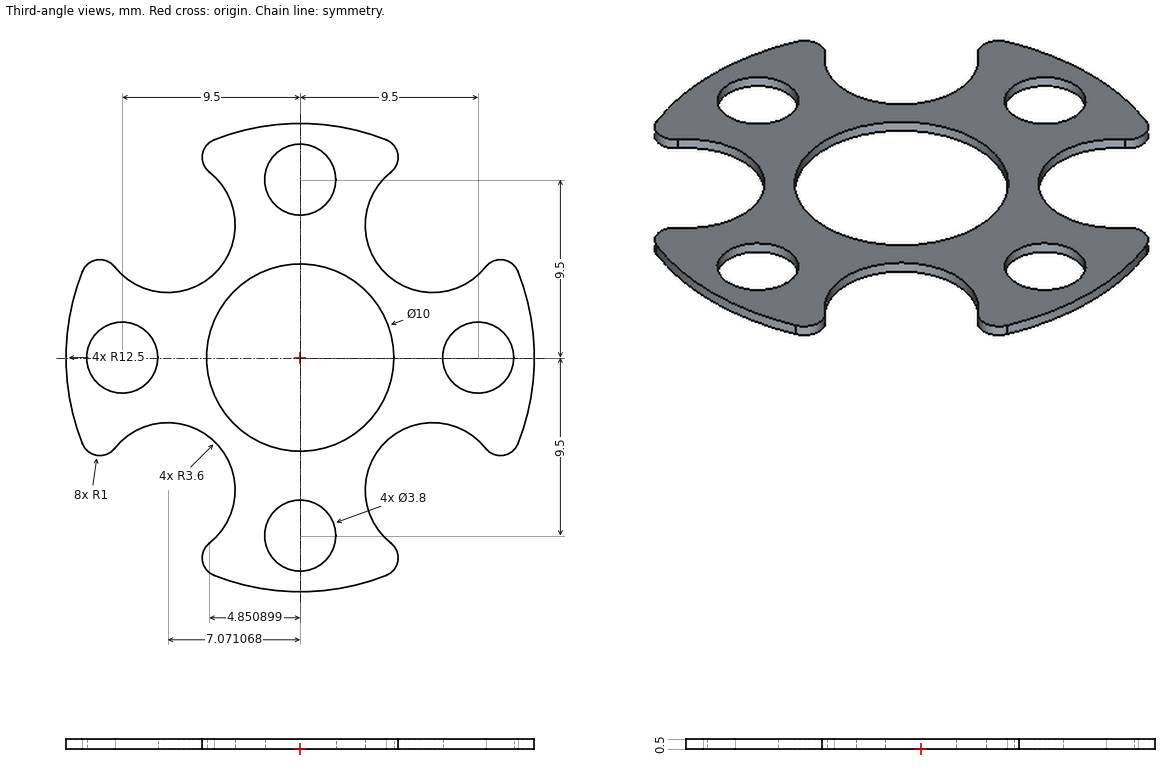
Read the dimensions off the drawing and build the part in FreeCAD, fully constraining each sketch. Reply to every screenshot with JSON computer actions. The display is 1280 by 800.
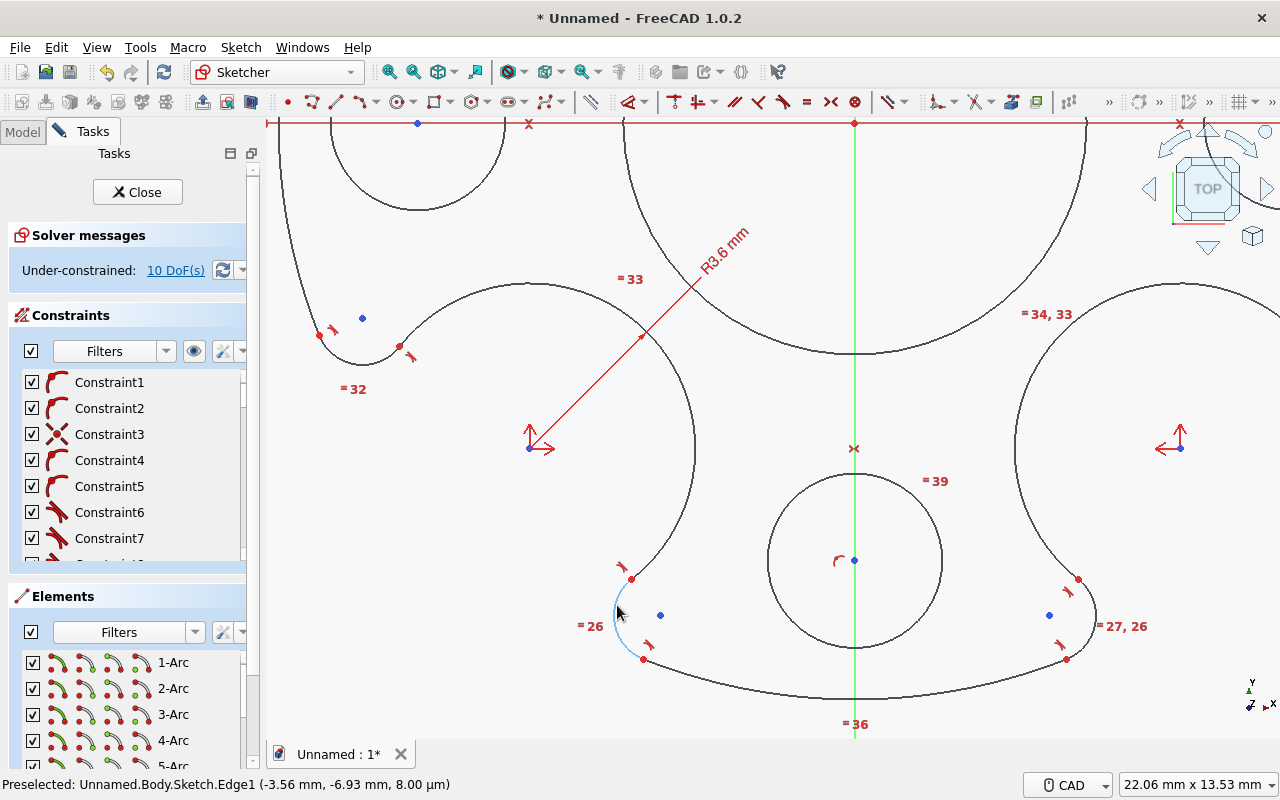
{"action": "left_click", "coordinate": [616, 603]}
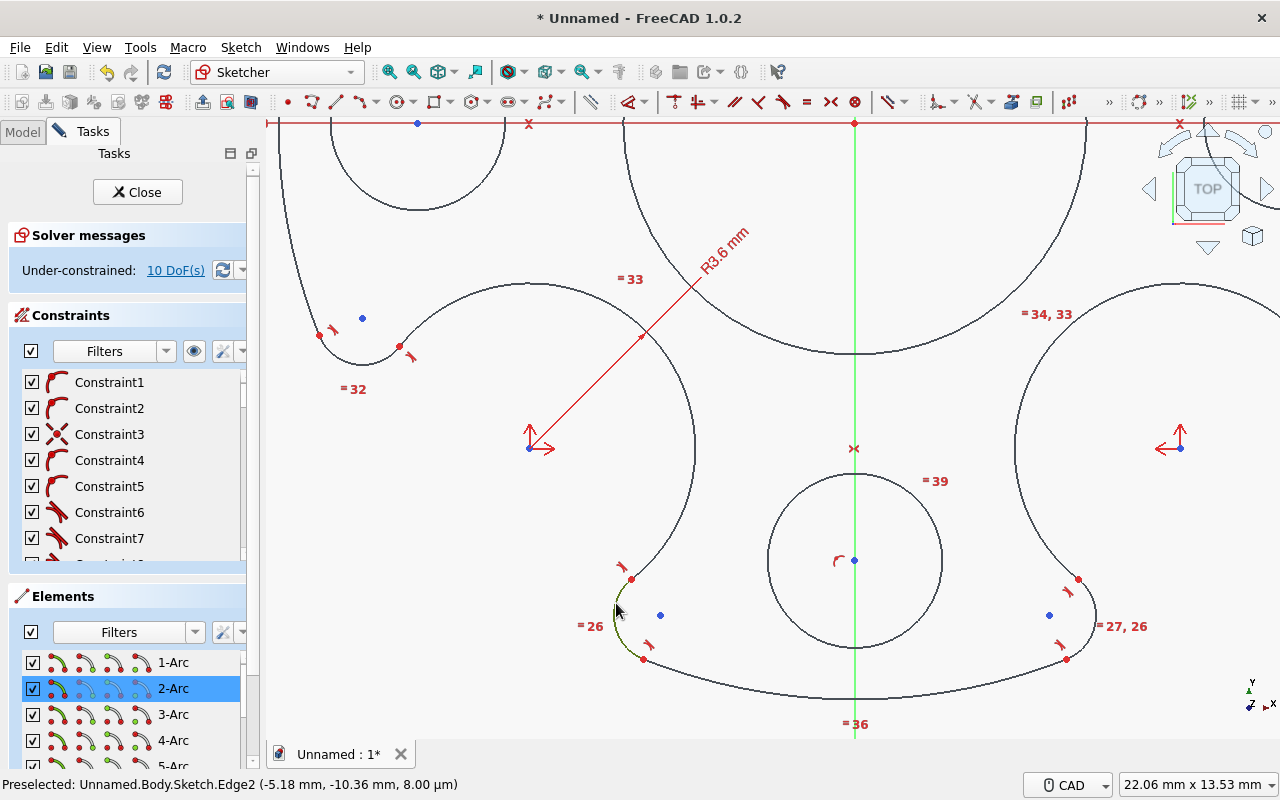
{"action": "key", "text": "k r"}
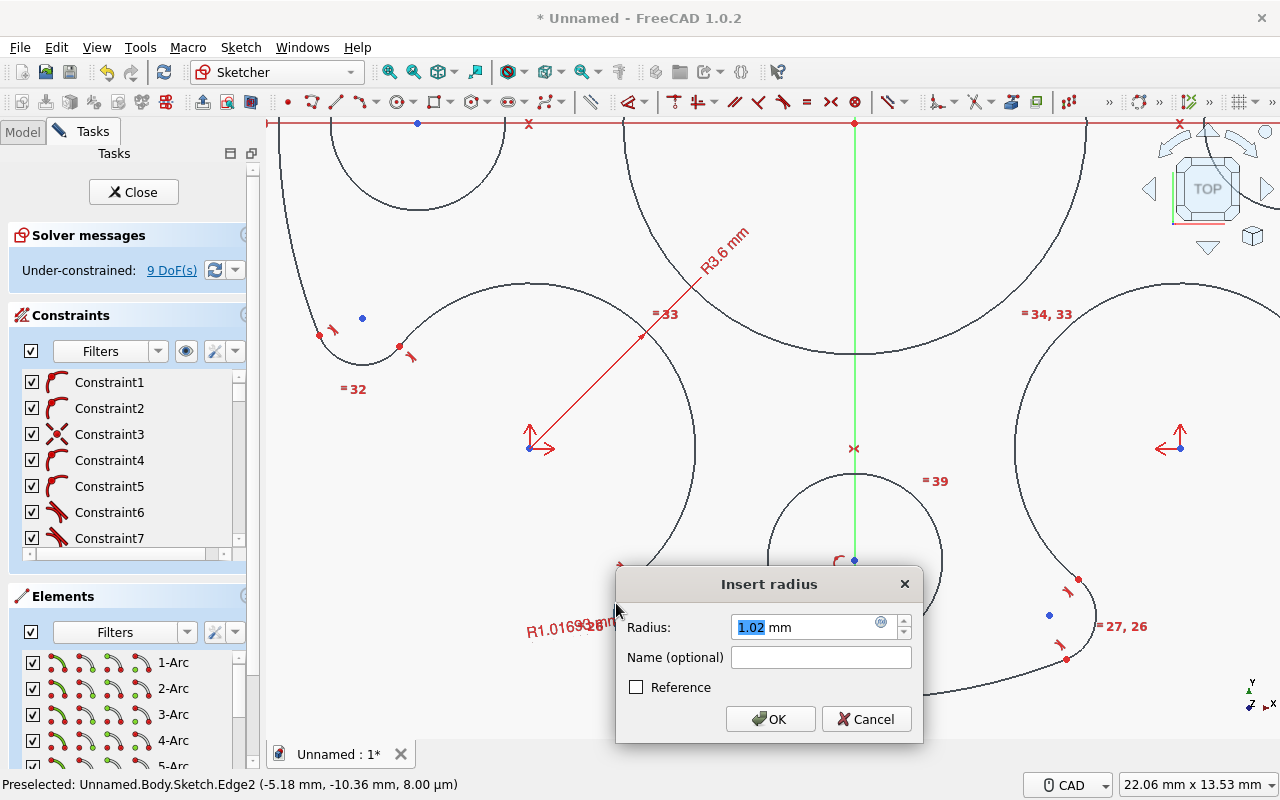
{"action": "type", "text": "1"}
{"action": "key", "text": "Return"}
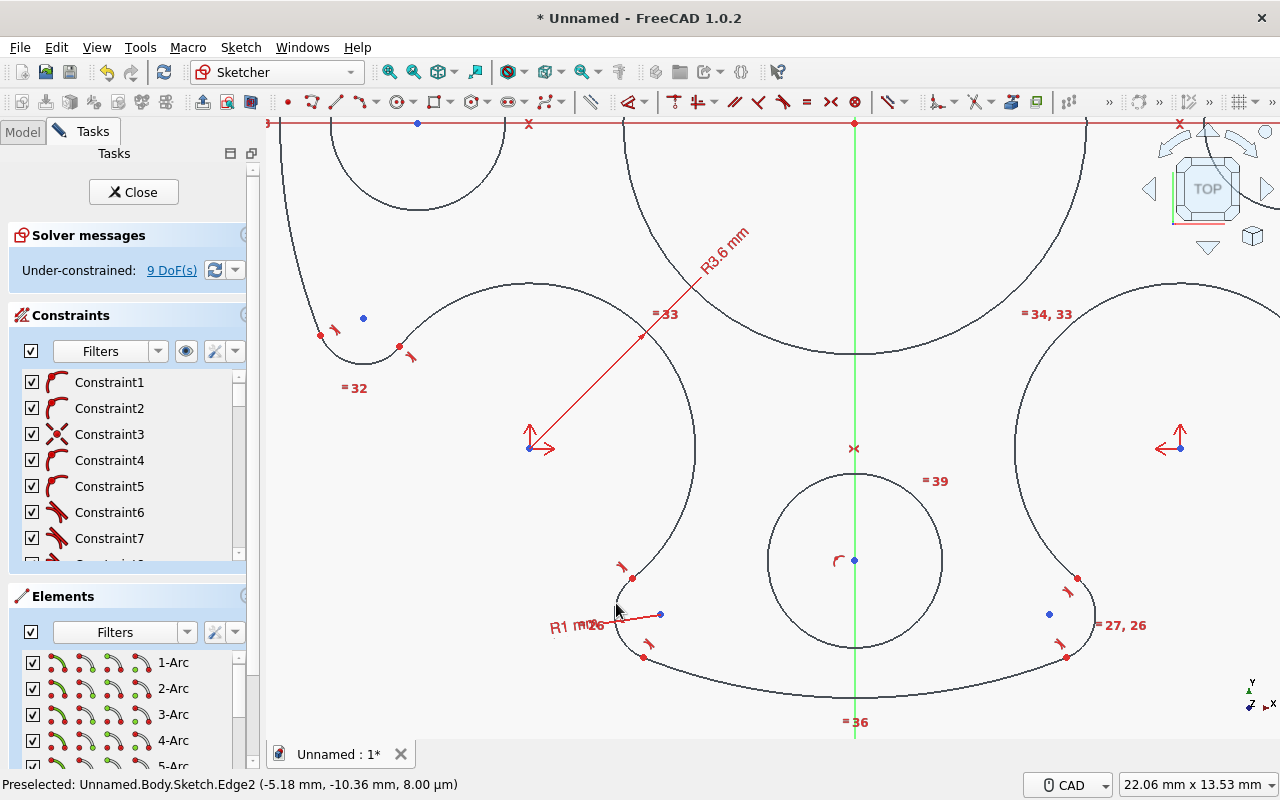
{"action": "left_click", "coordinate": [769, 691]}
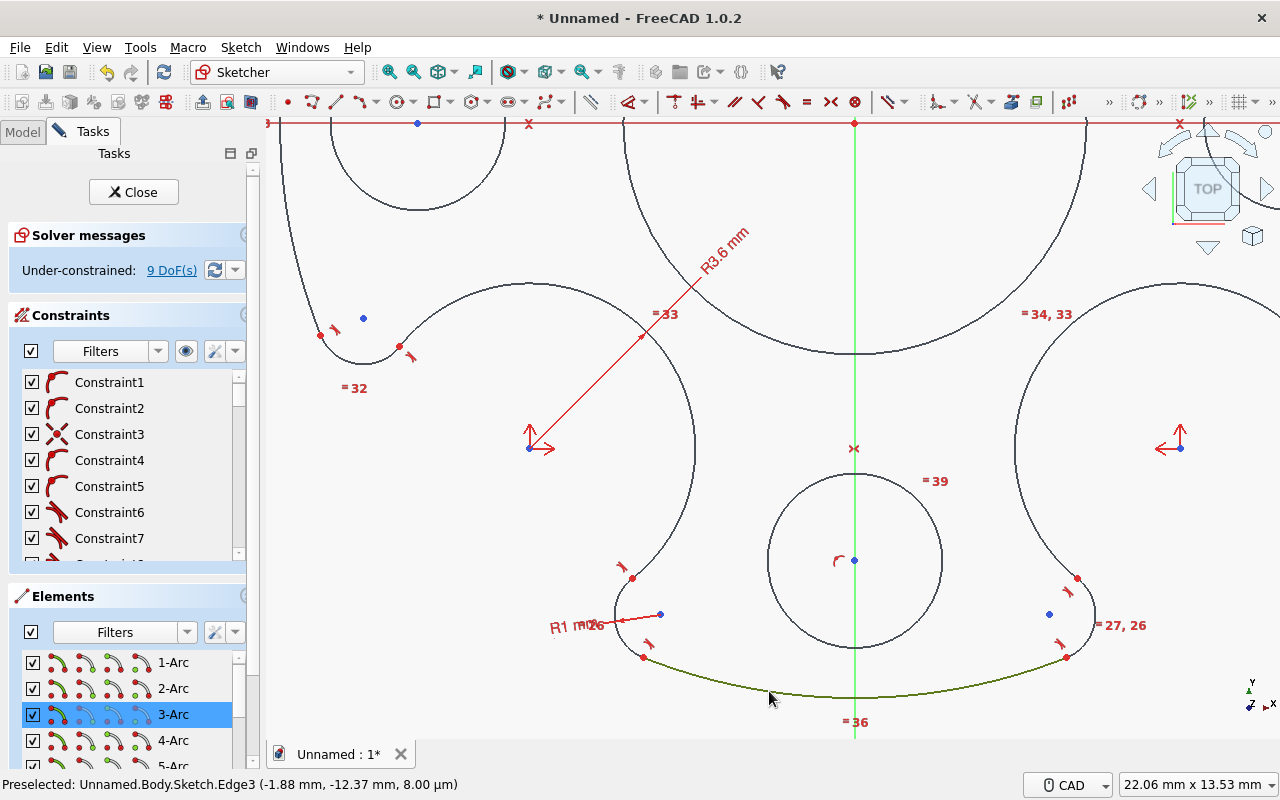
{"action": "key", "text": "k r"}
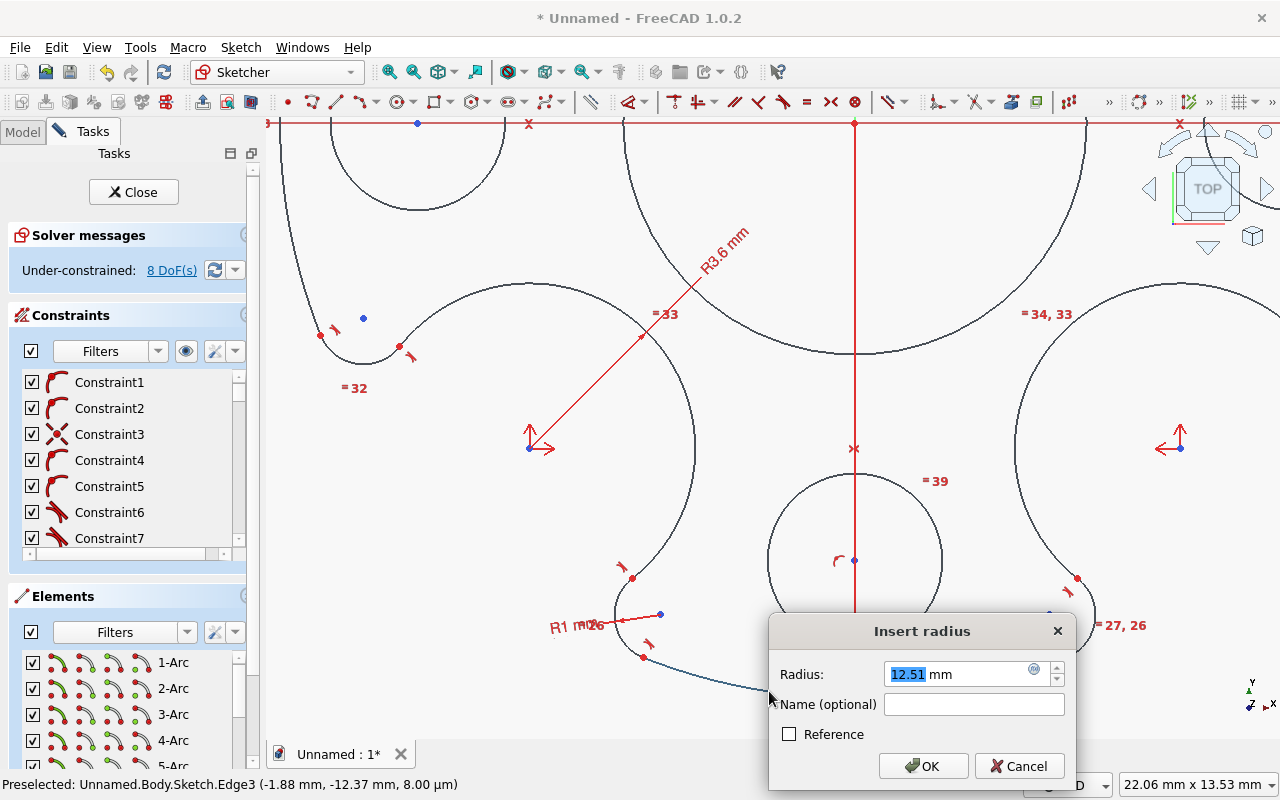
{"action": "type", "text": "12.5"}
{"action": "key", "text": "Return"}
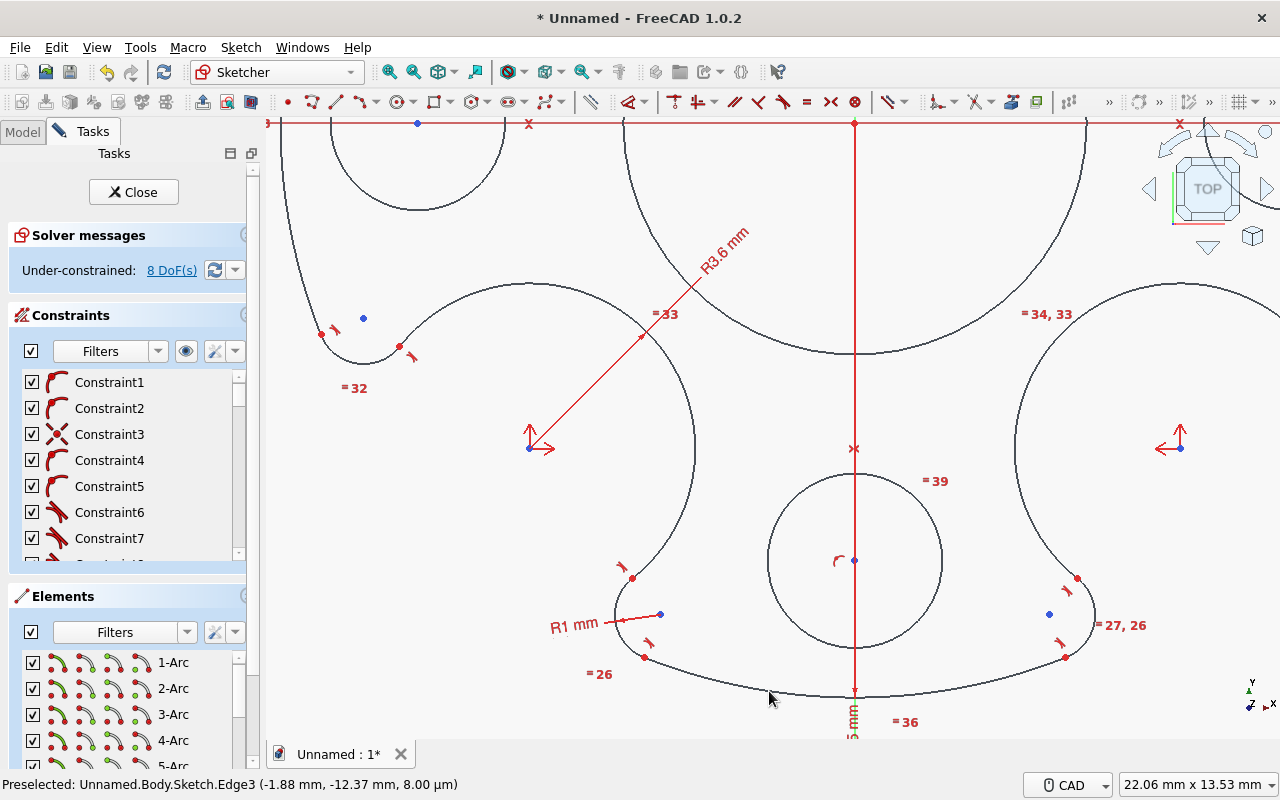
{"action": "left_click", "coordinate": [917, 499]}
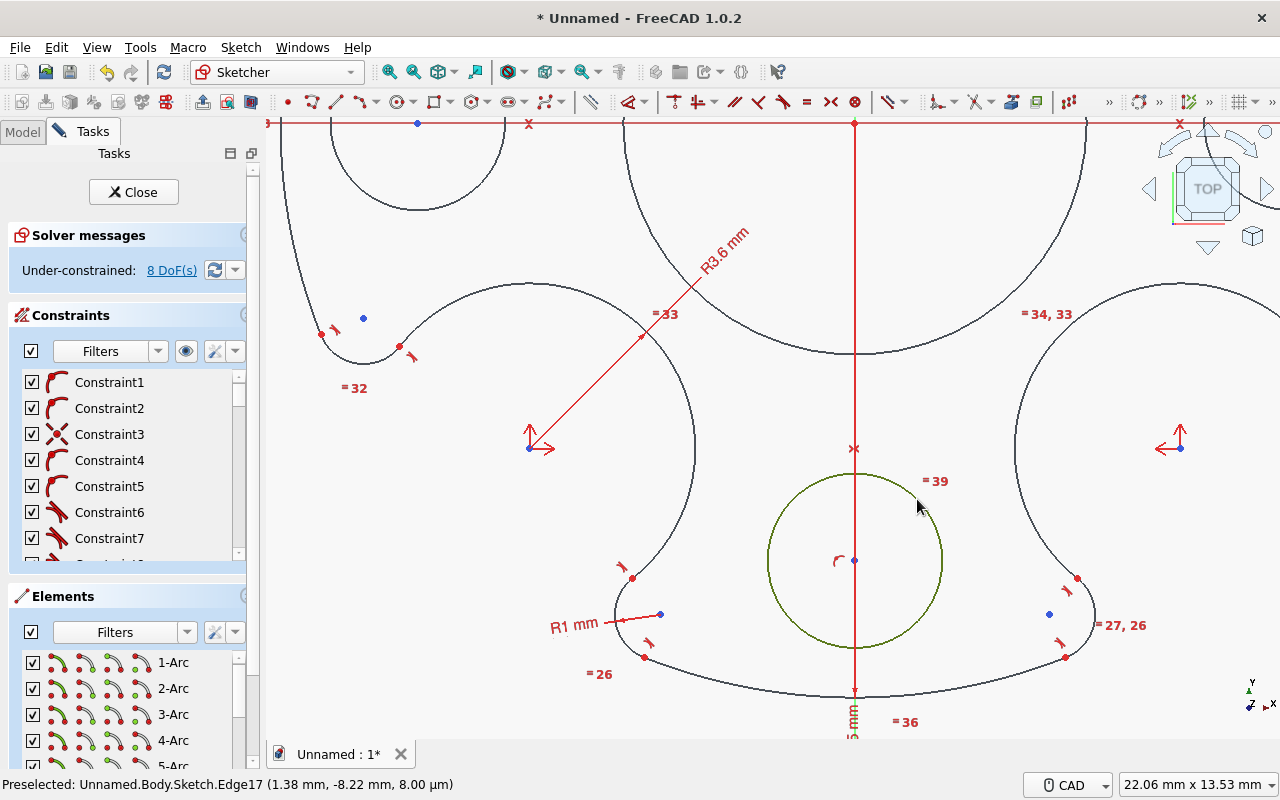
{"action": "key", "text": "k o"}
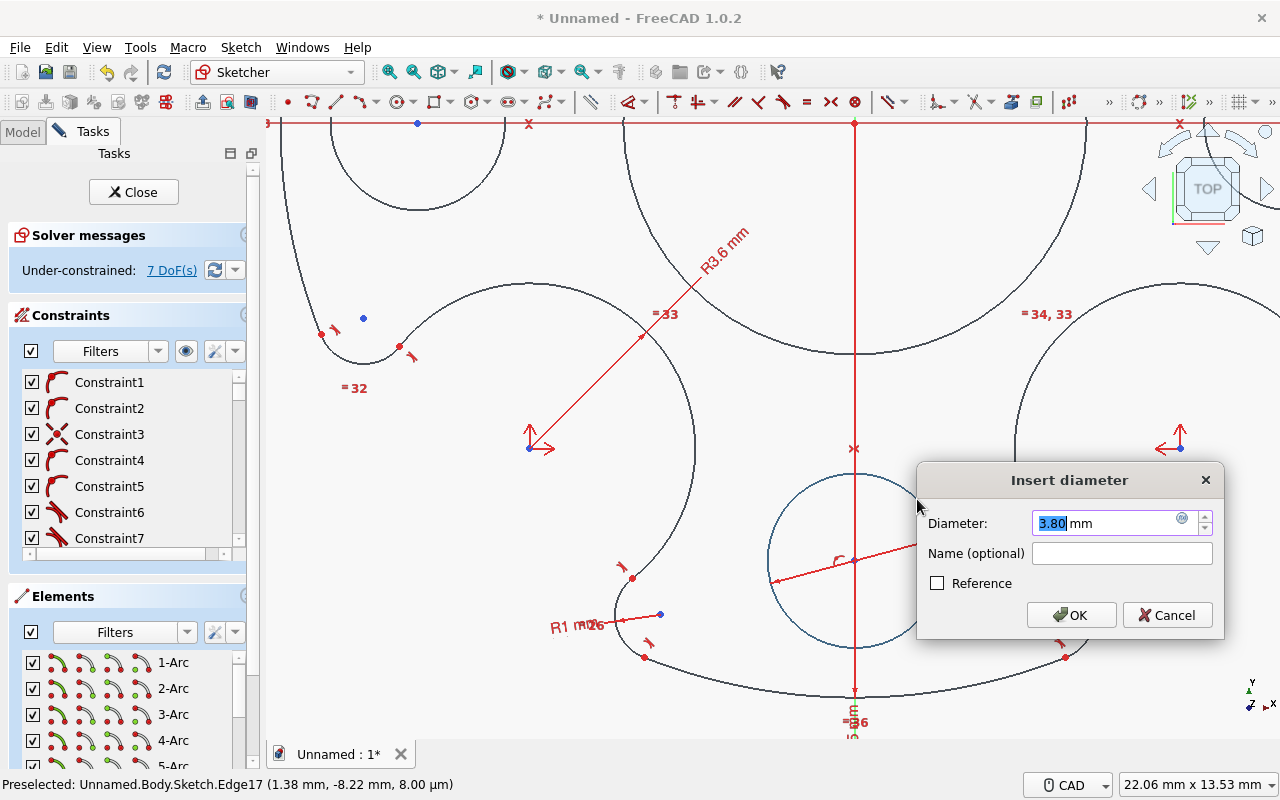
{"action": "type", "text": "3.8"}
{"action": "key", "text": "Return"}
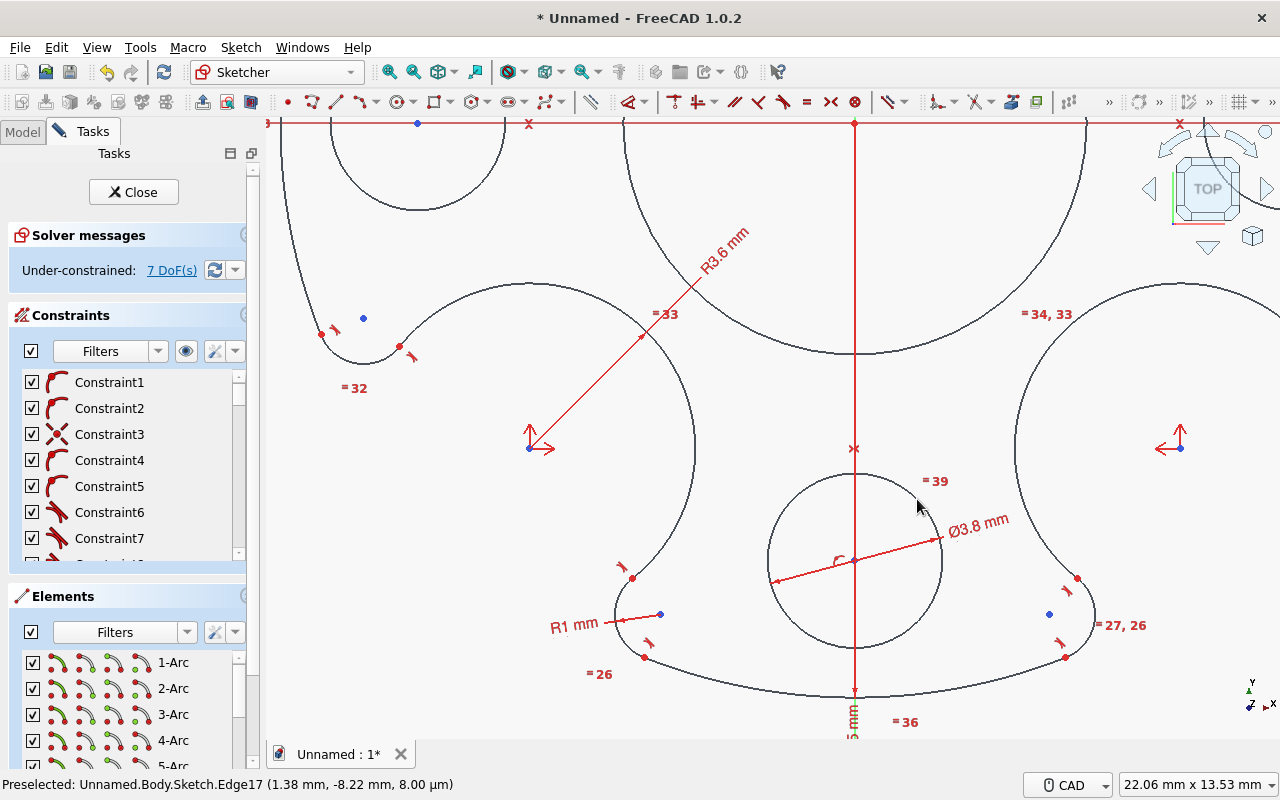
{"action": "left_click", "coordinate": [692, 287]}